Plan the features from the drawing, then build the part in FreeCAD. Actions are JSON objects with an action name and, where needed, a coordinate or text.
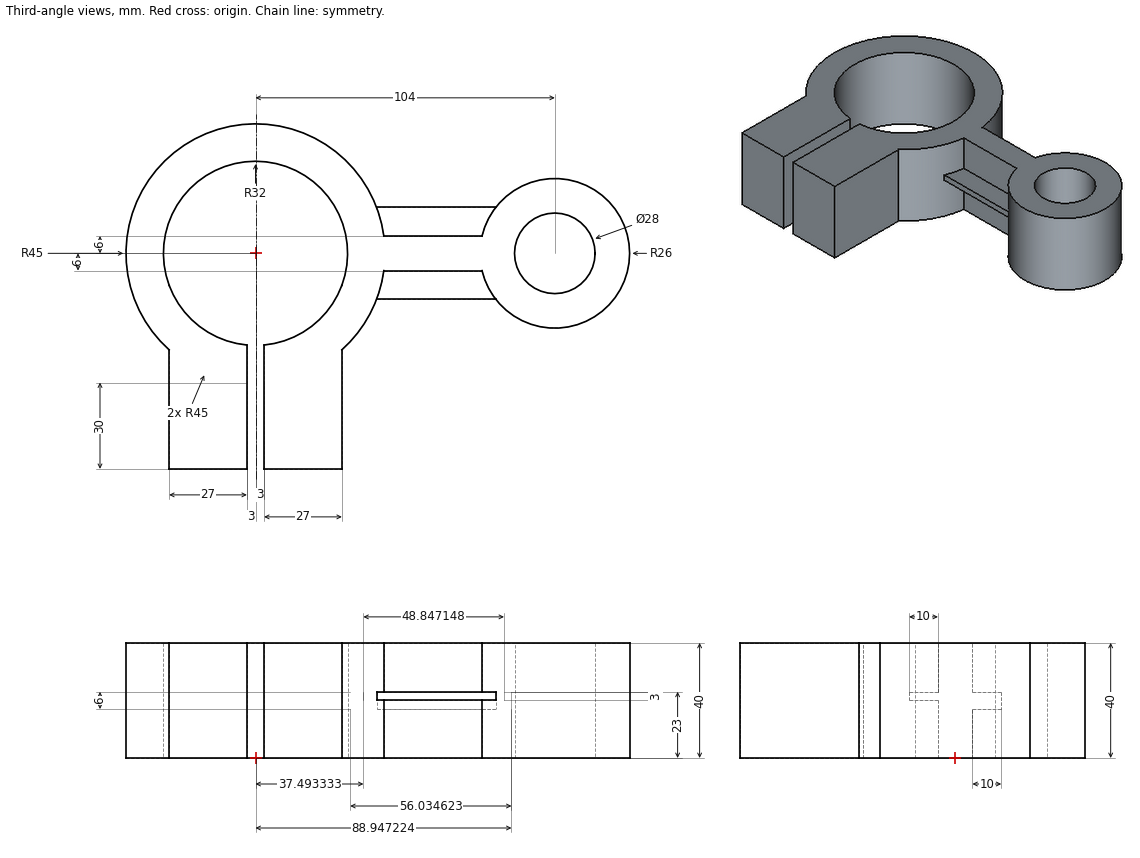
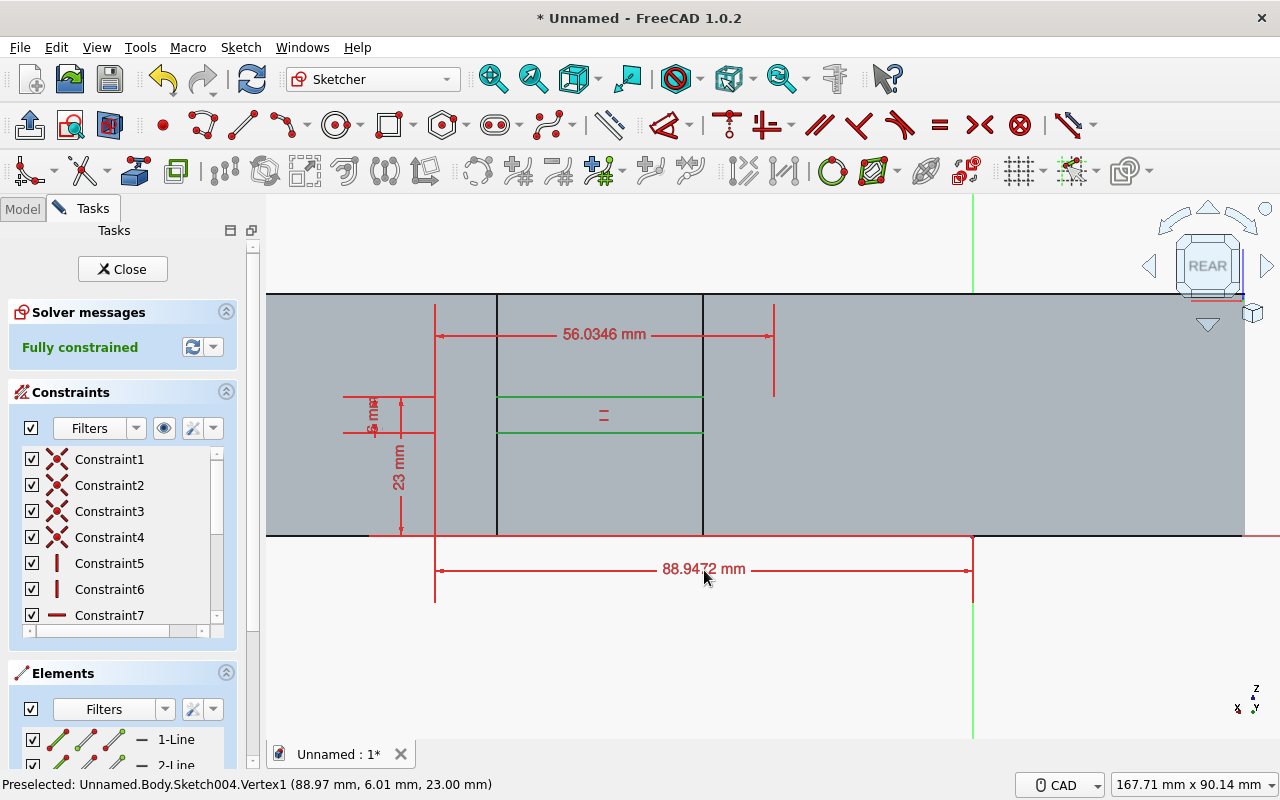
{"action": "left_click", "coordinate": [123, 269]}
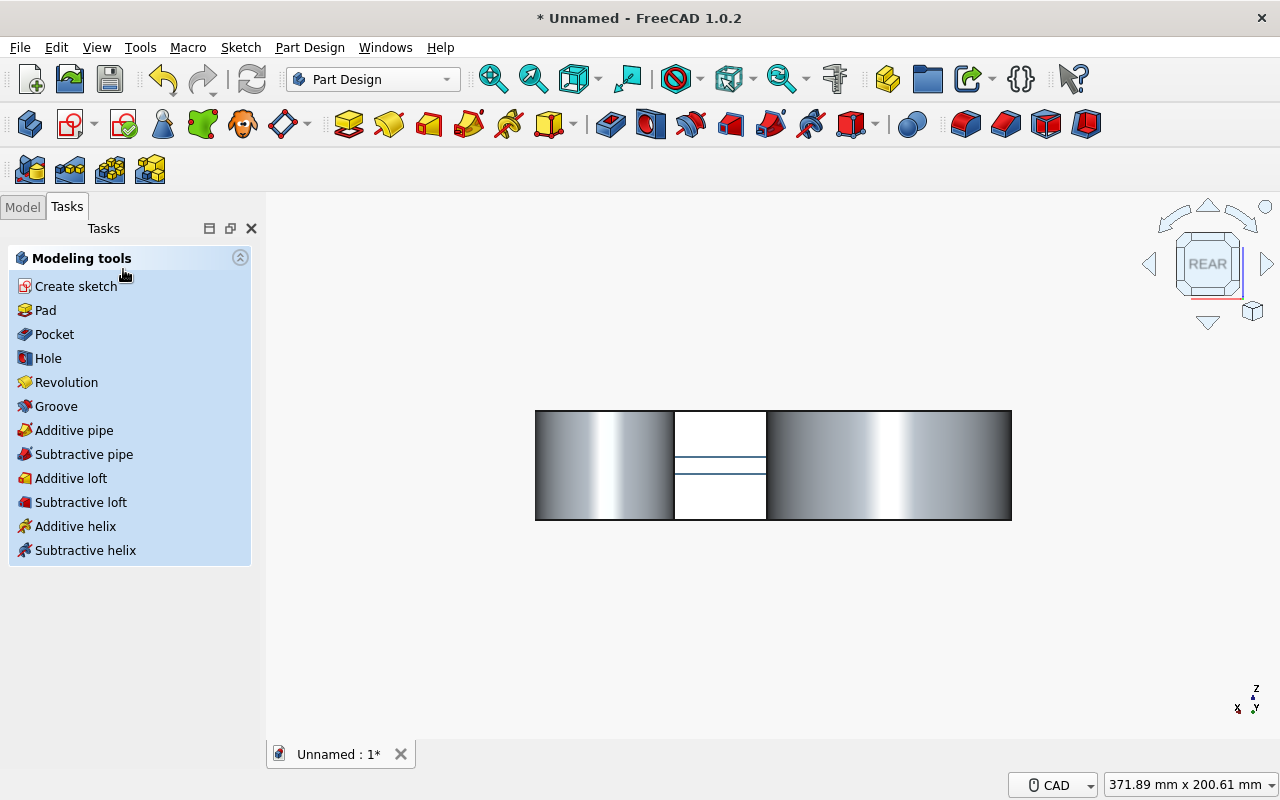
{"action": "left_click", "coordinate": [350, 124]}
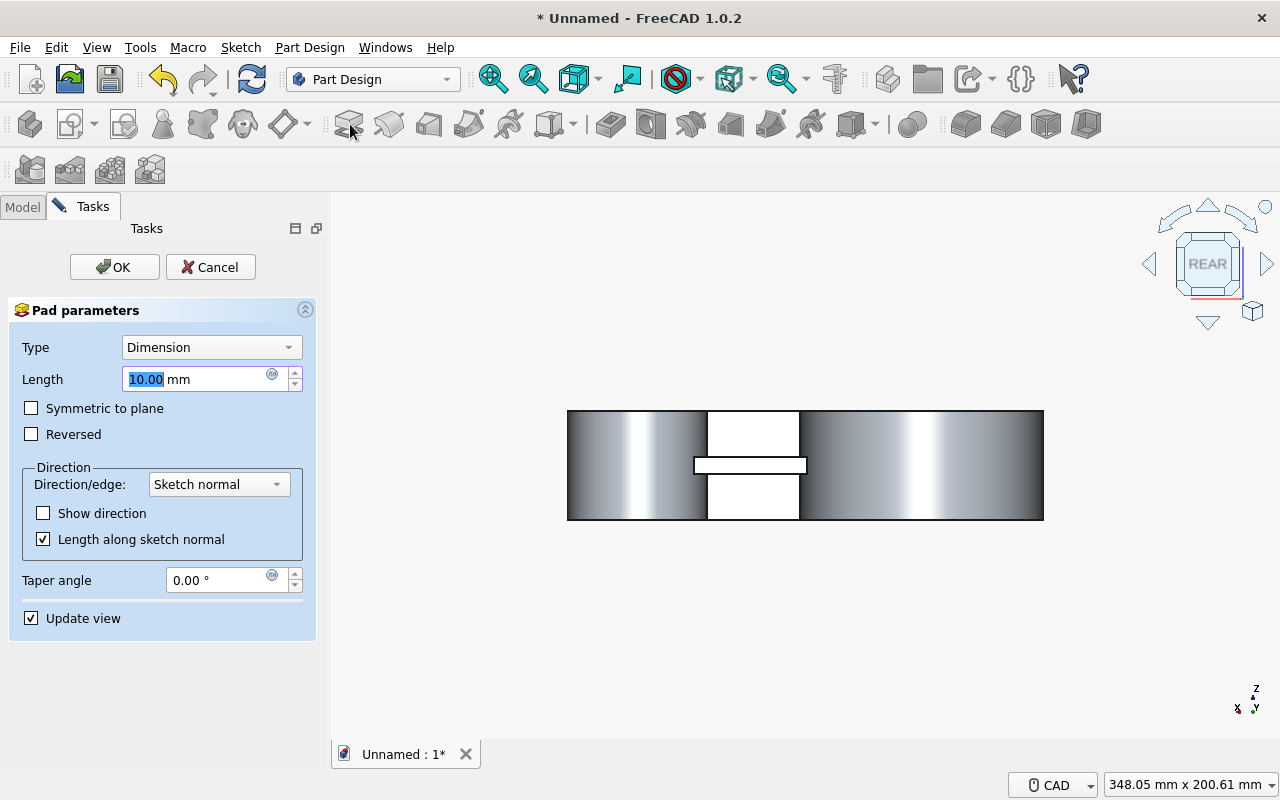
{"action": "type", "text": "10"}
{"action": "key", "text": "Tab"}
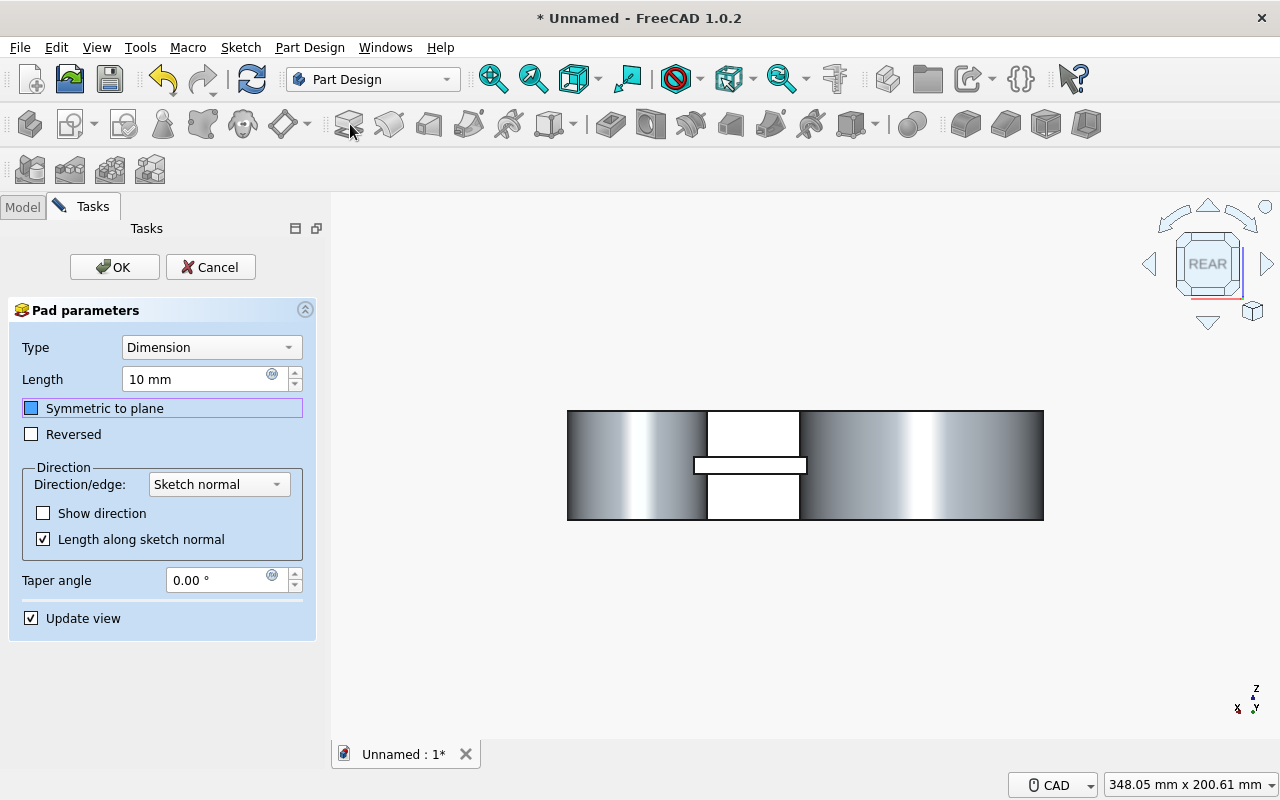
{"action": "left_click", "coordinate": [115, 267]}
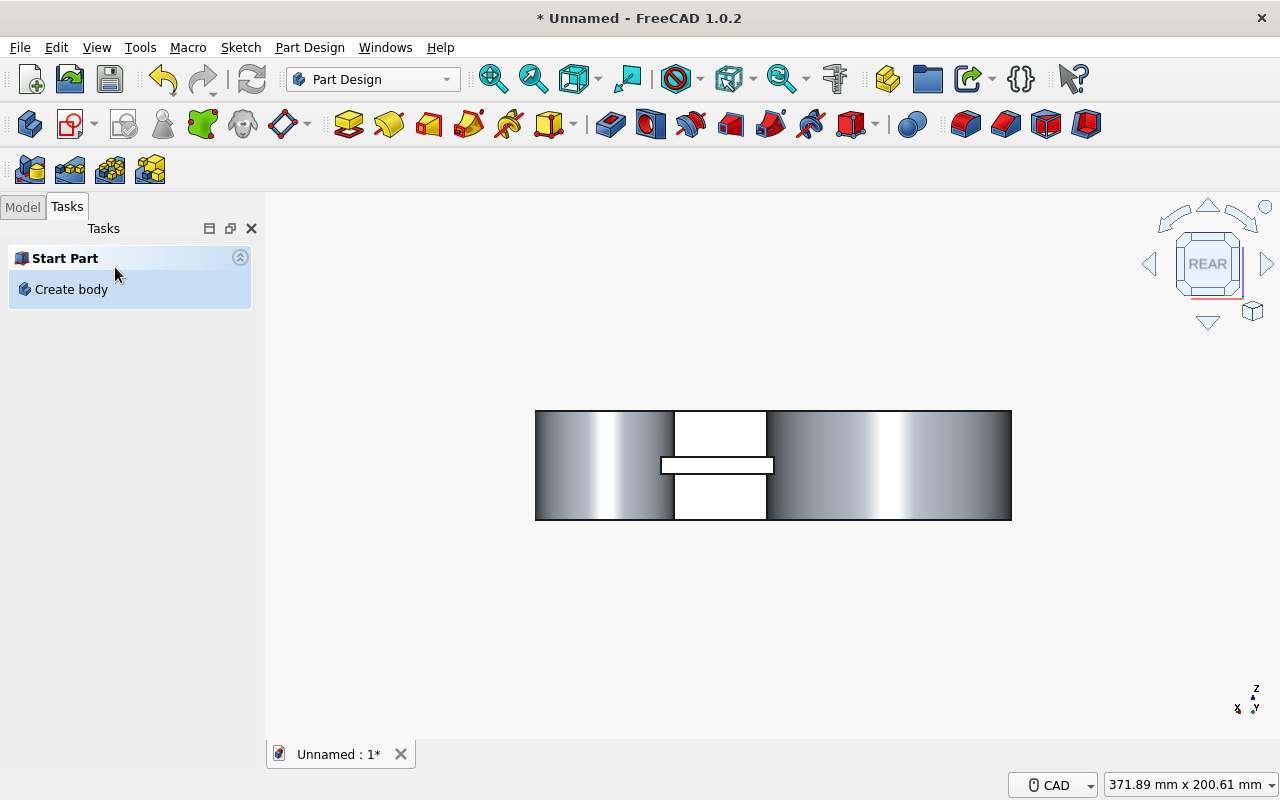
{"action": "key", "text": "0"}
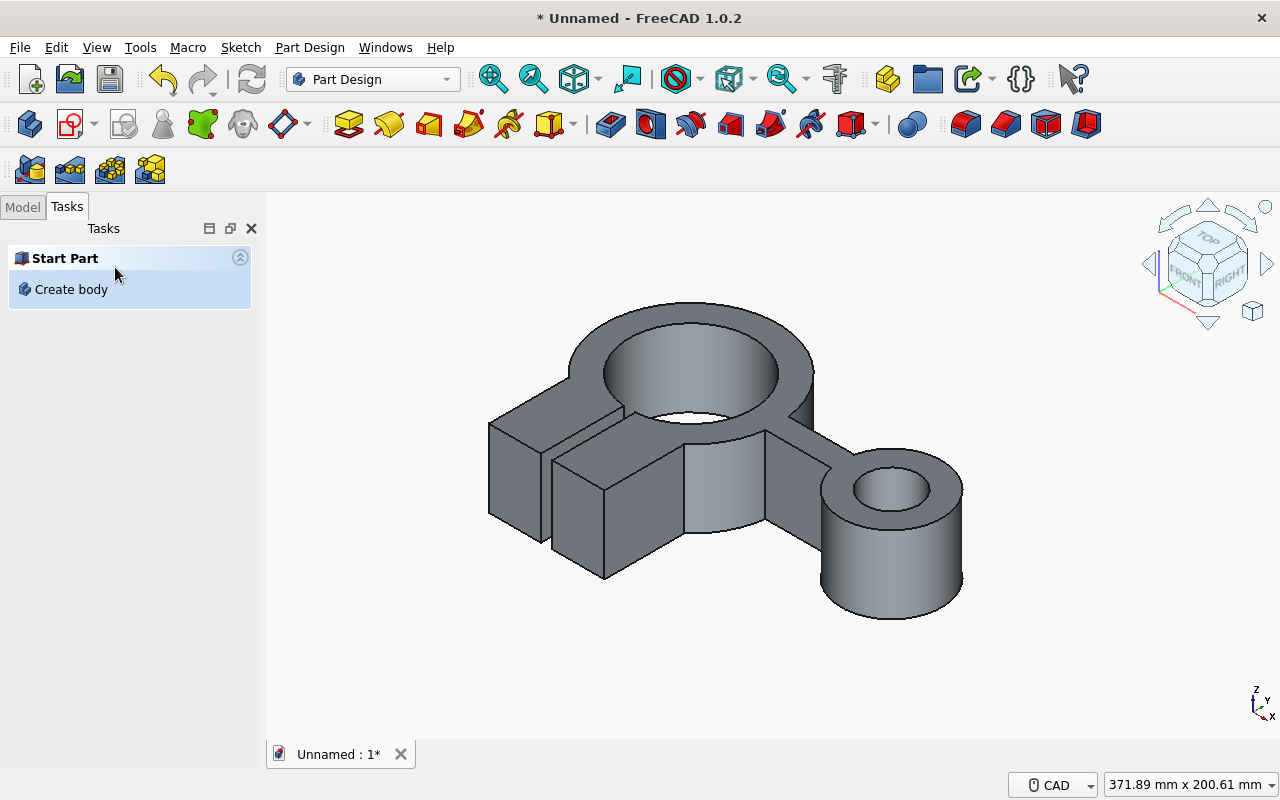
{"action": "left_click", "coordinate": [798, 492]}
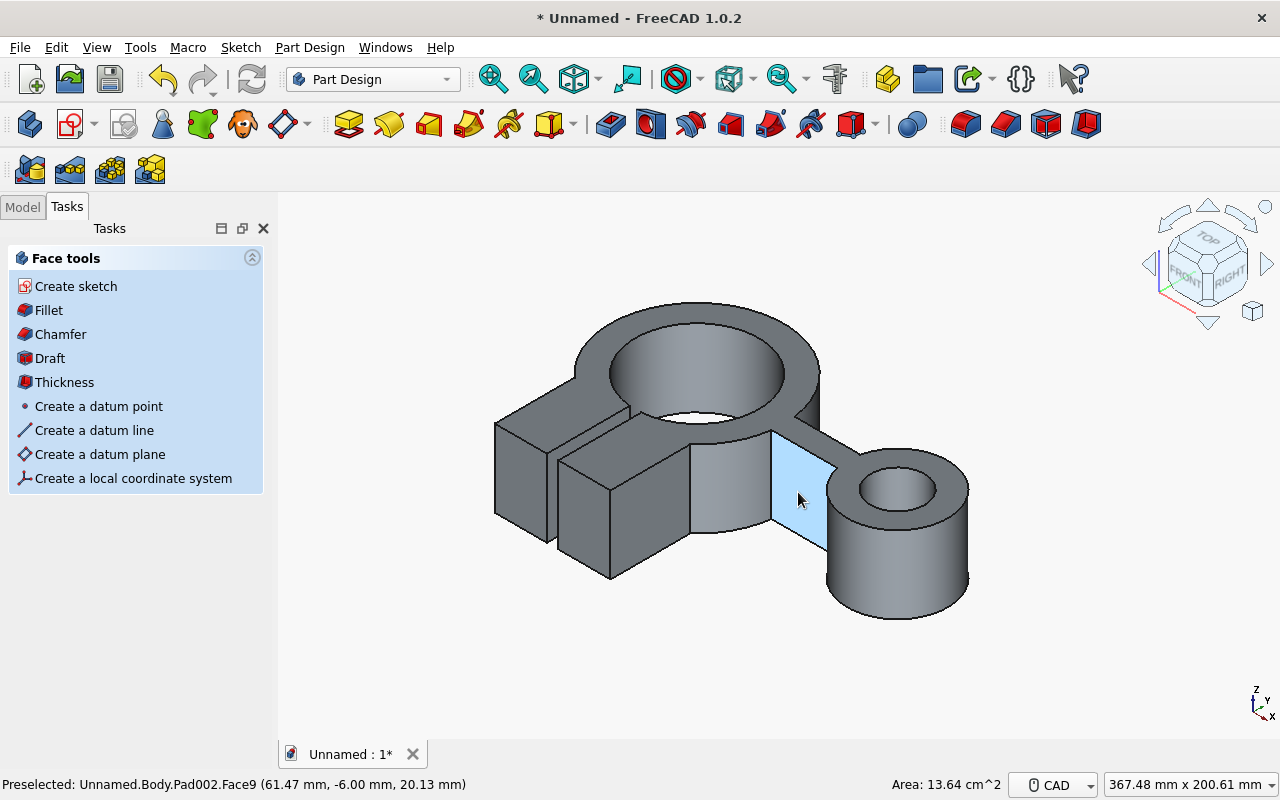
{"action": "left_click", "coordinate": [70, 124]}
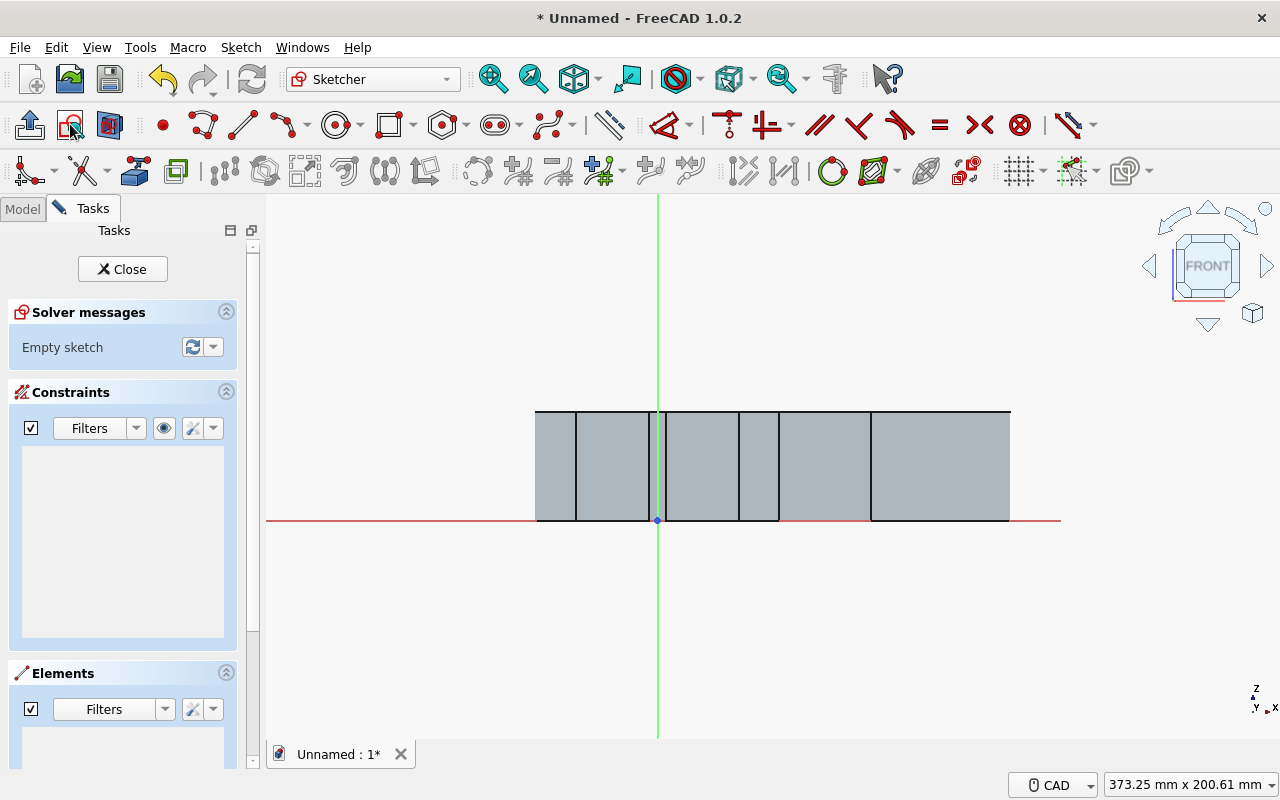
{"action": "key", "text": "q s"}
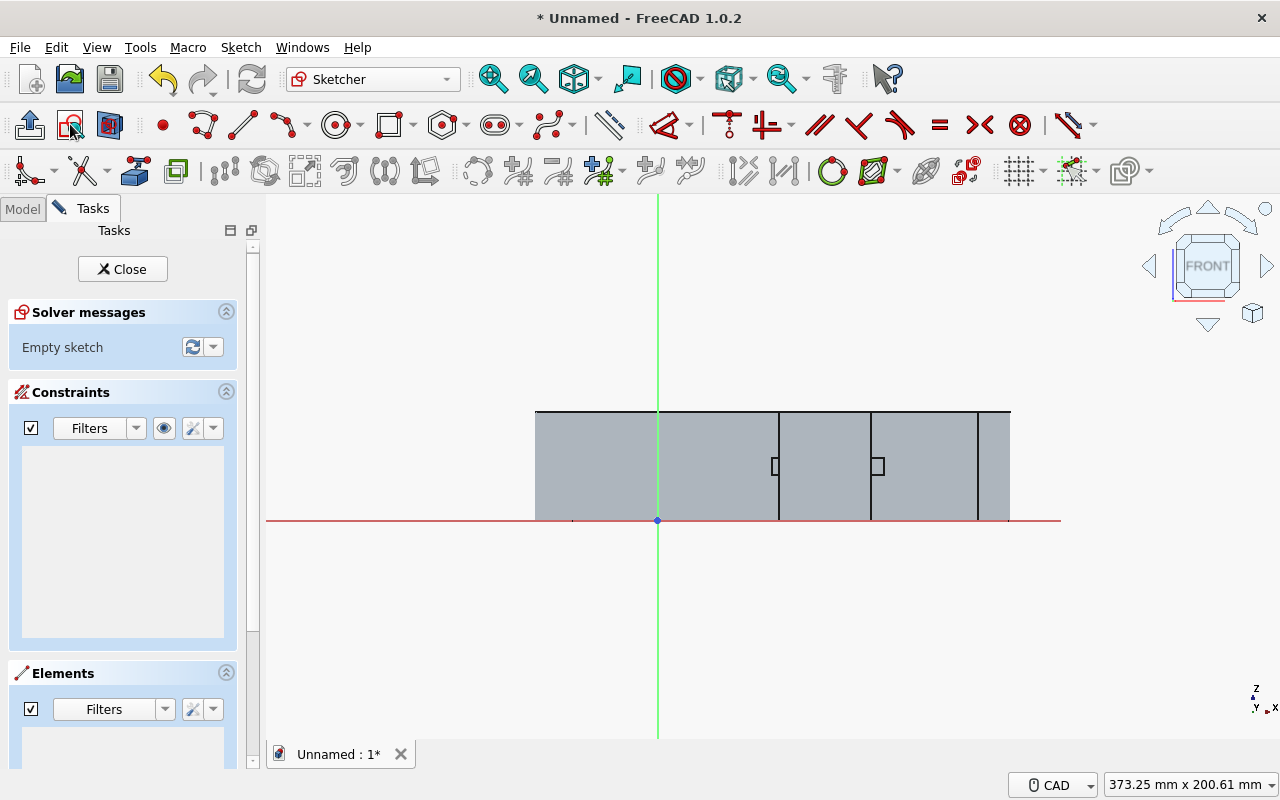
{"action": "scroll", "coordinate": [816, 503], "scroll_direction": "up", "scroll_amount": 5}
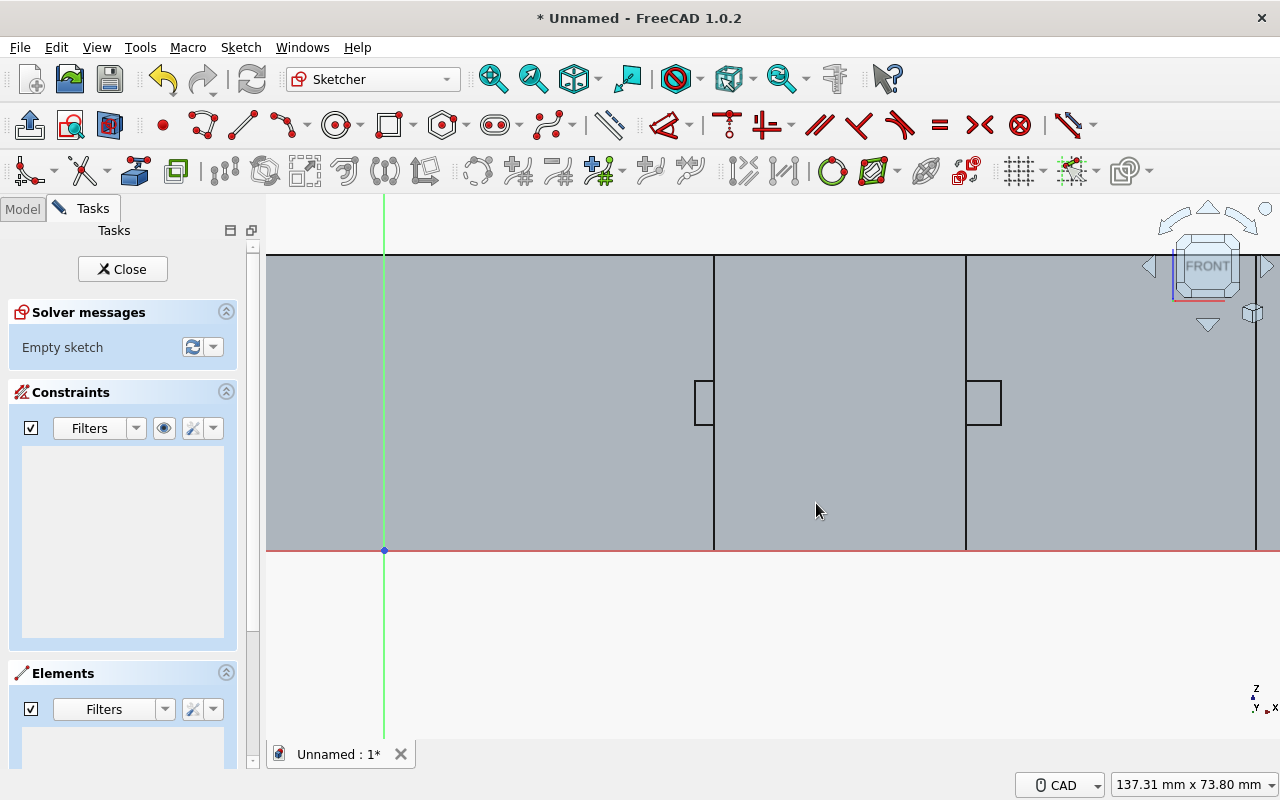
{"action": "key", "text": "g r"}